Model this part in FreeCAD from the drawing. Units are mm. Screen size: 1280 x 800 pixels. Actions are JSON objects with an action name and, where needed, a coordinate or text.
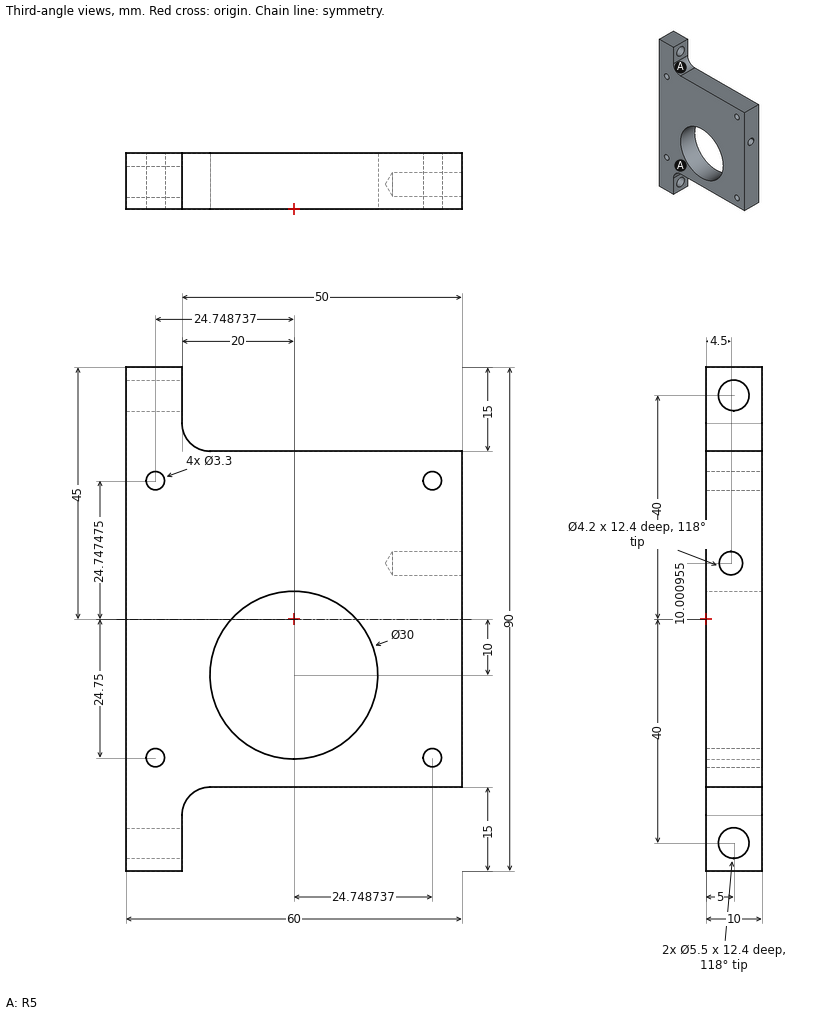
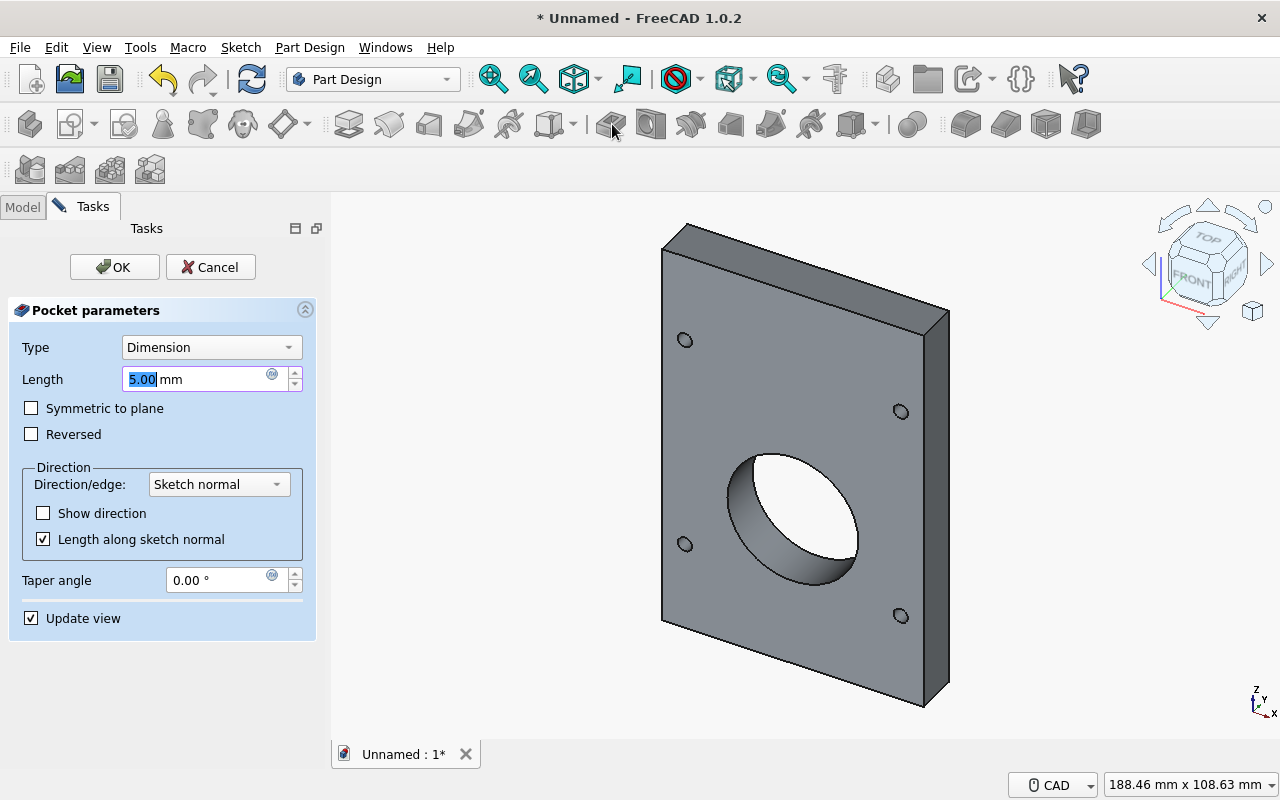
{"action": "left_click", "coordinate": [212, 348]}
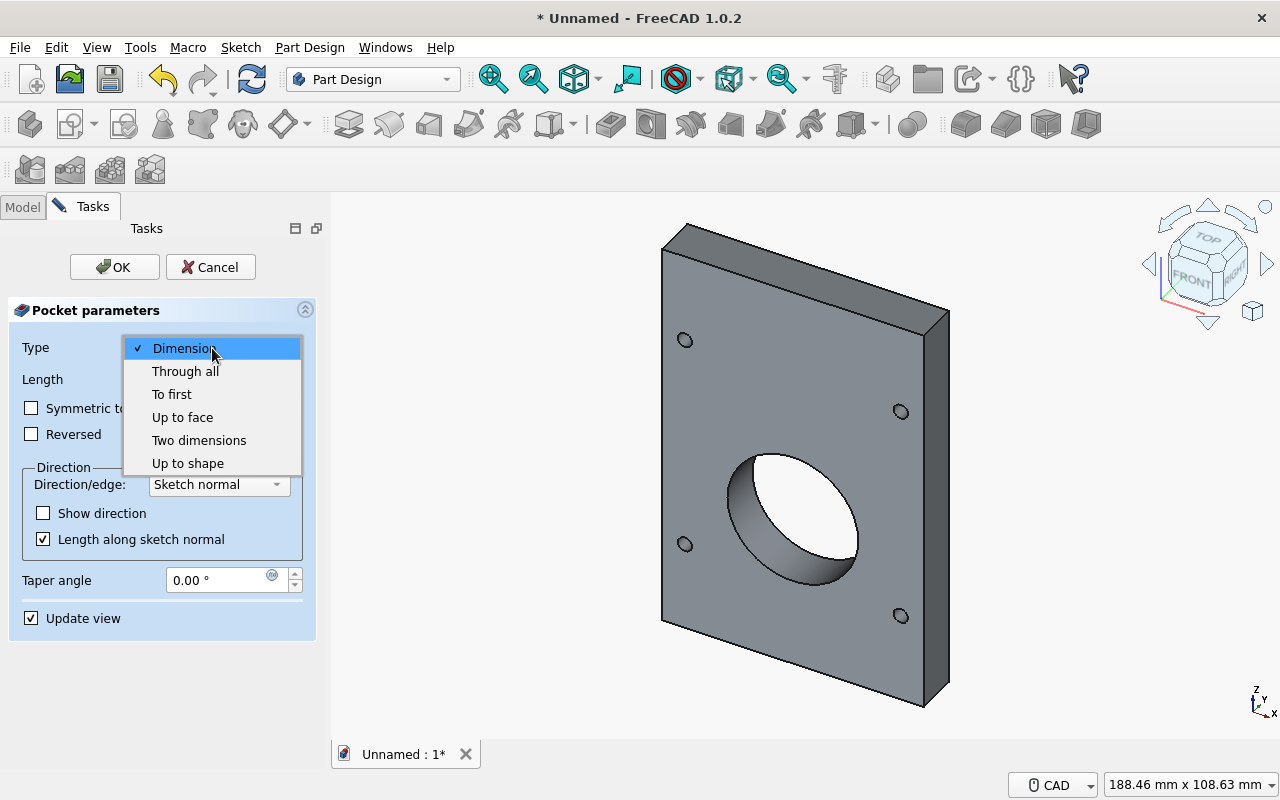
{"action": "left_click", "coordinate": [212, 372]}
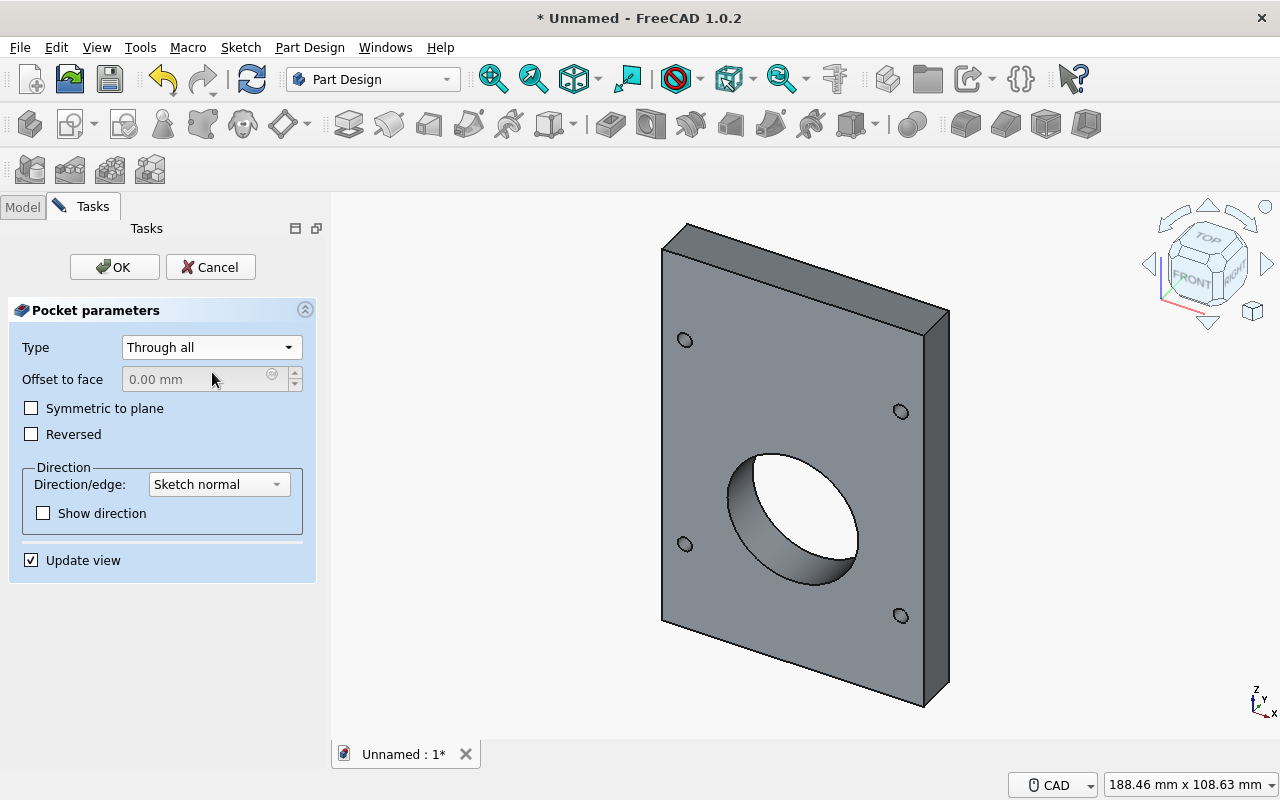
{"action": "left_click", "coordinate": [115, 267]}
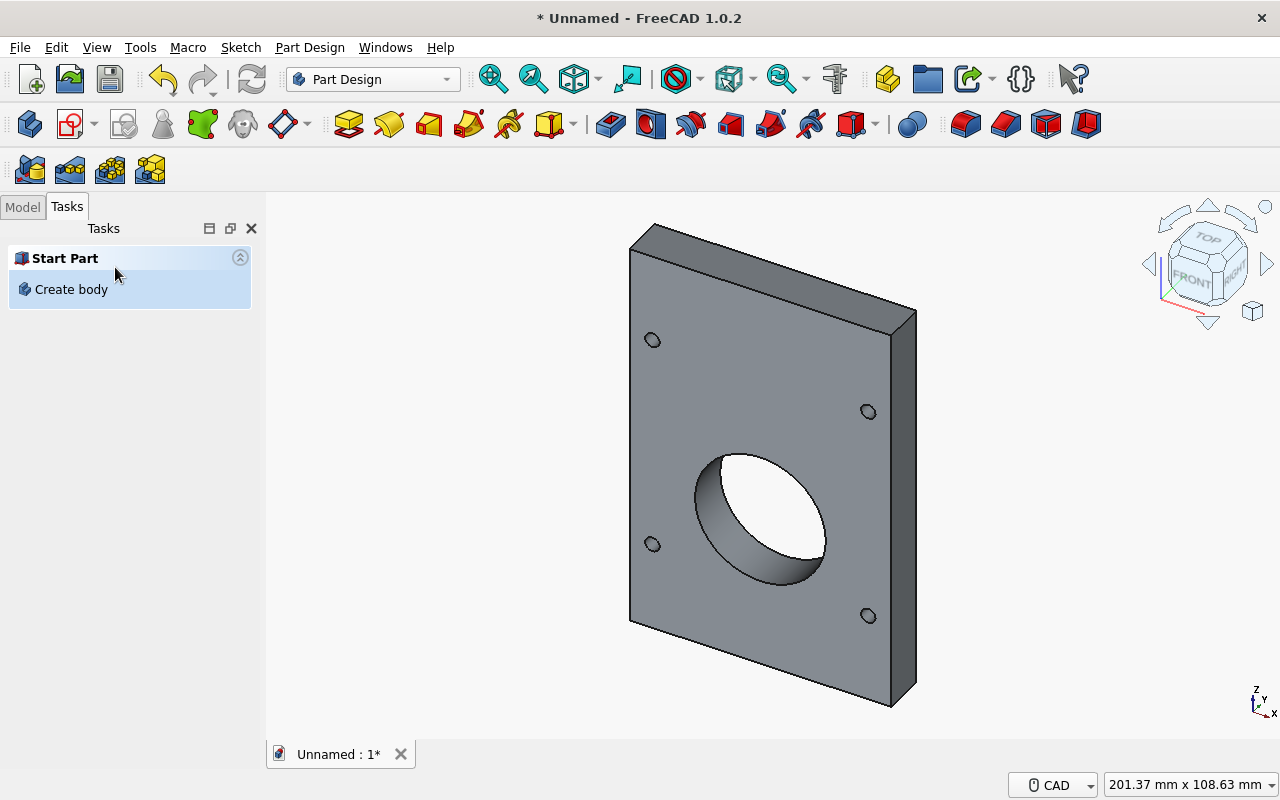
{"action": "left_click", "coordinate": [760, 371]}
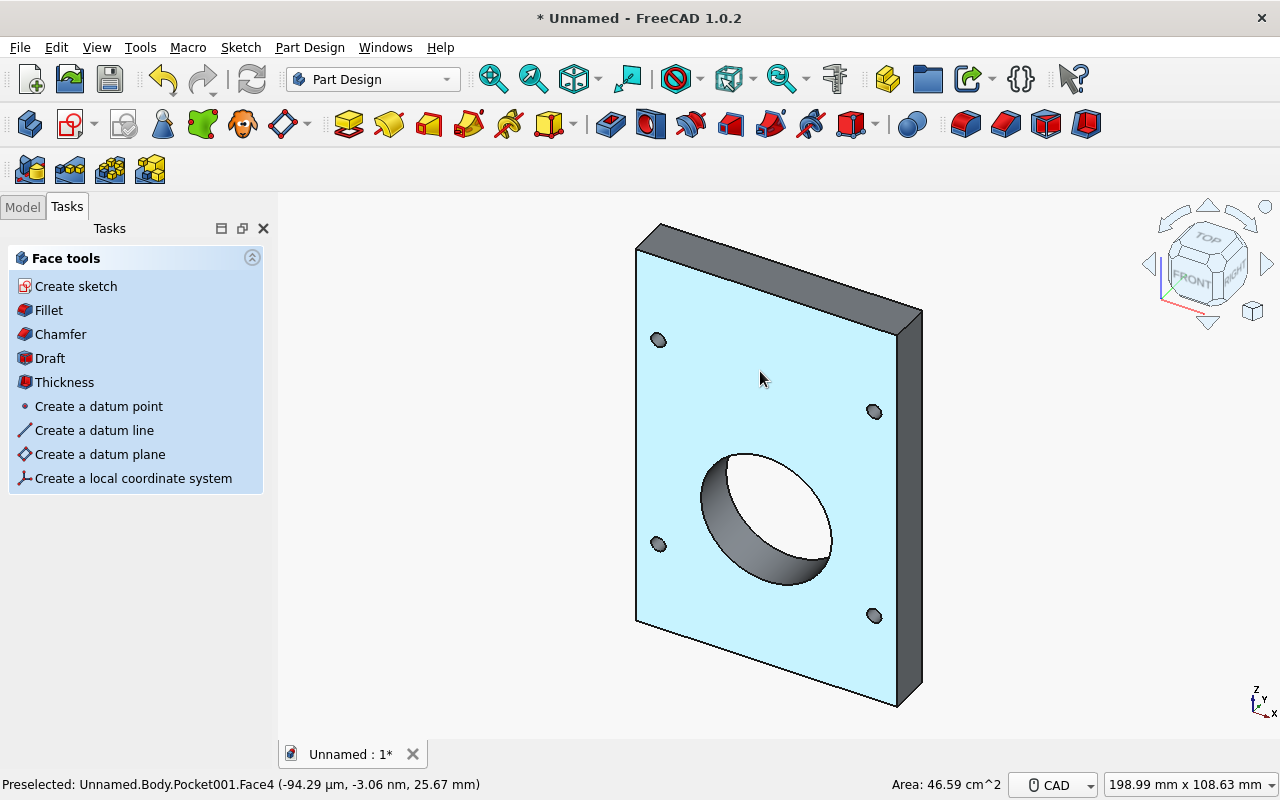
{"action": "left_click", "coordinate": [70, 124]}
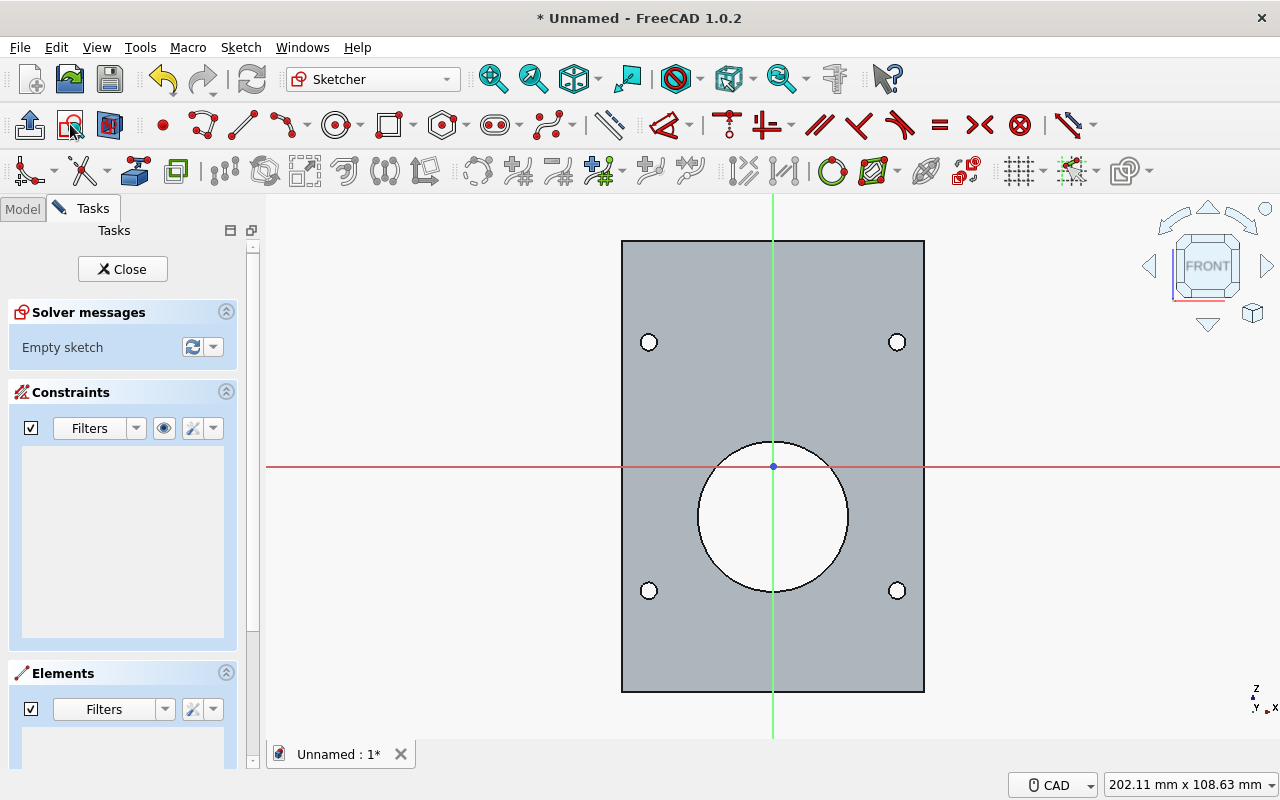
{"action": "scroll", "coordinate": [294, 466], "scroll_direction": "down", "scroll_amount": 1}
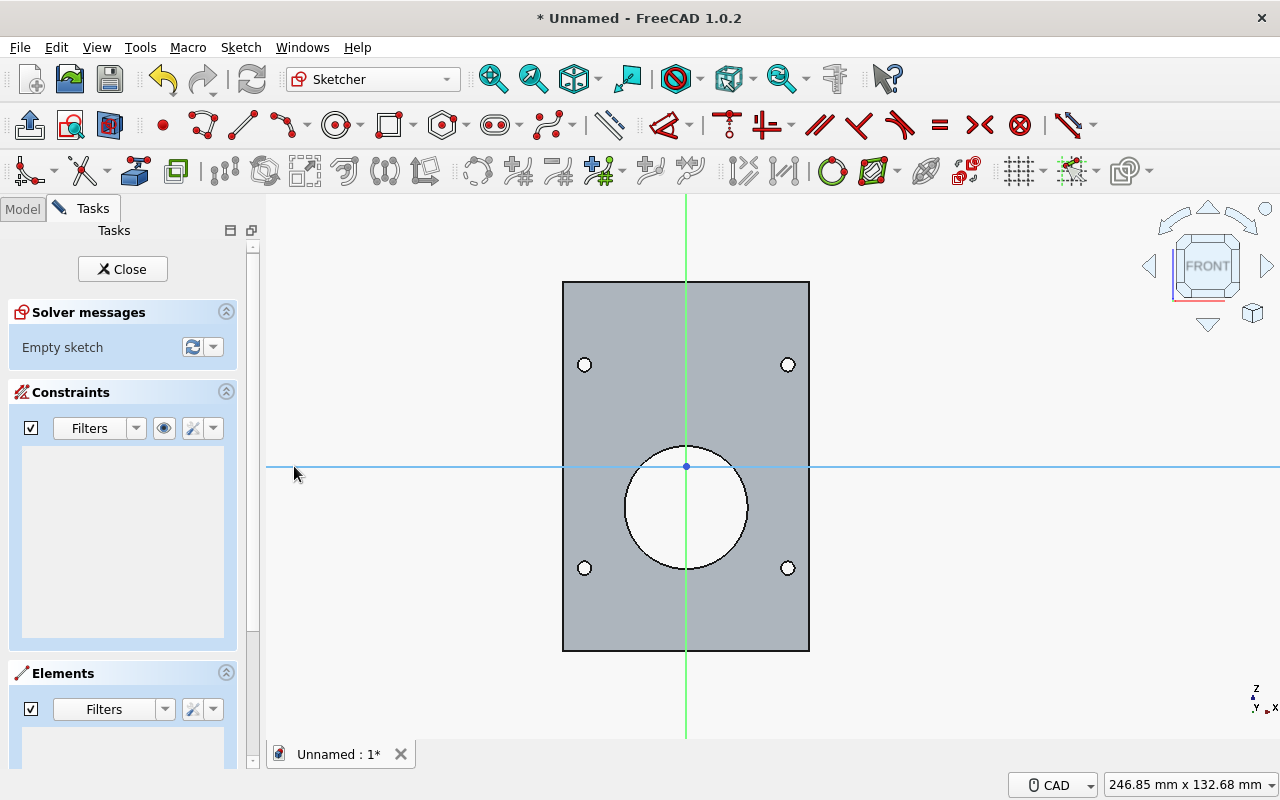
{"action": "left_click", "coordinate": [390, 126]}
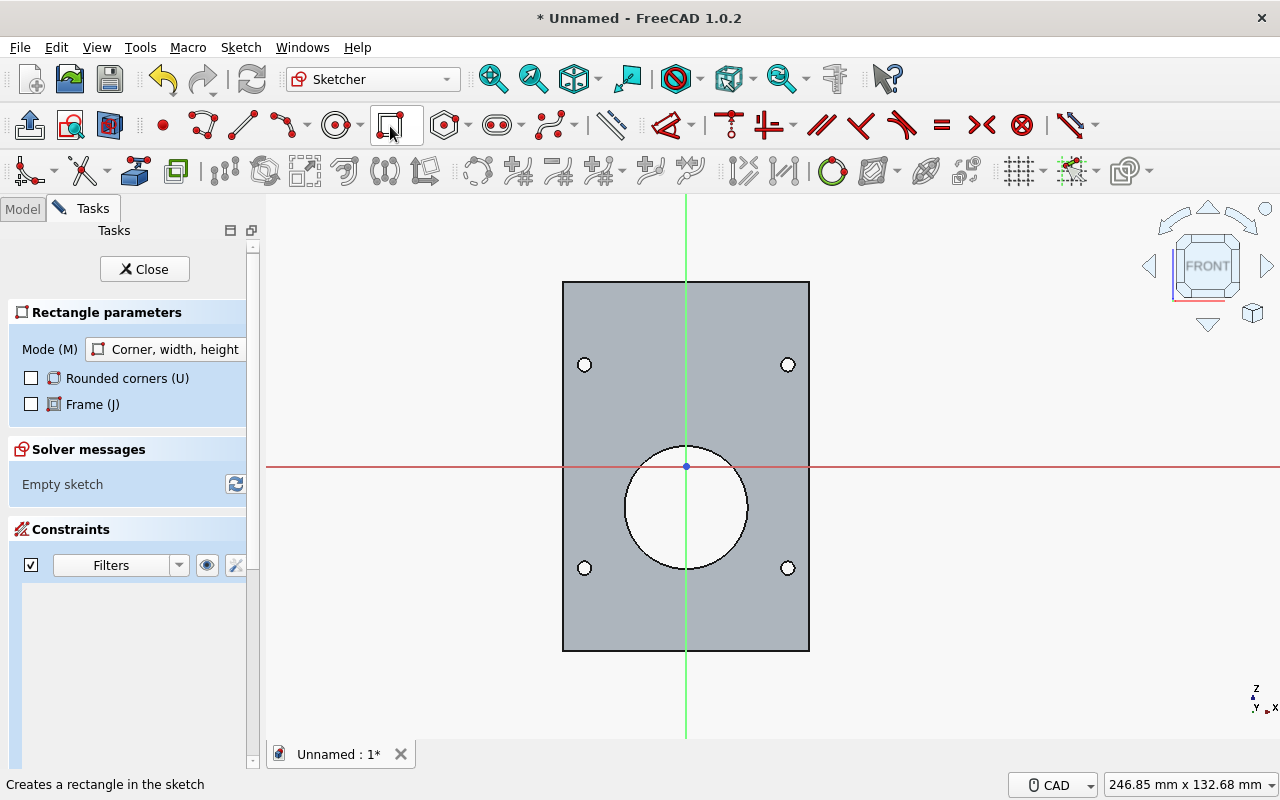
{"action": "left_click", "coordinate": [604, 282]}
{"action": "mouse_move", "coordinate": [809, 343]}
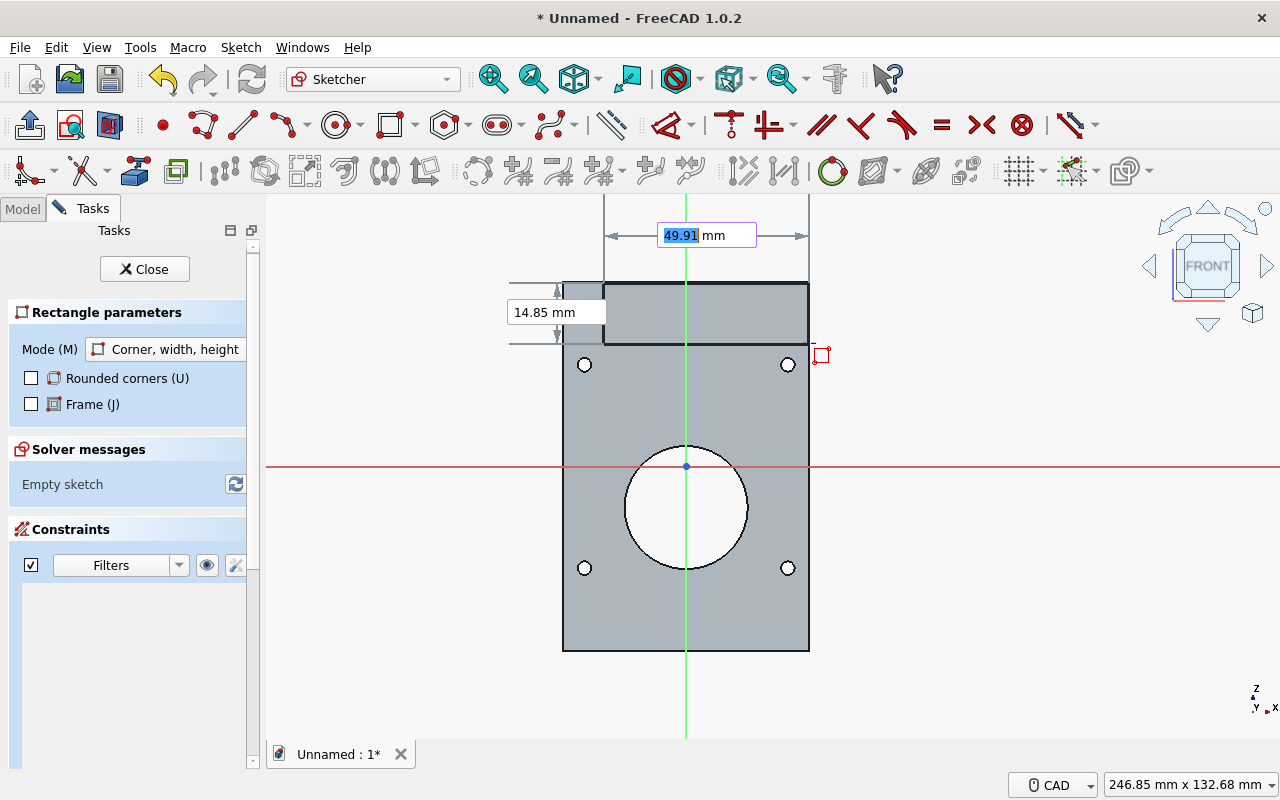
{"action": "type", "text": "50"}
{"action": "key", "text": "Tab"}
{"action": "type", "text": "15"}
{"action": "key", "text": "Return"}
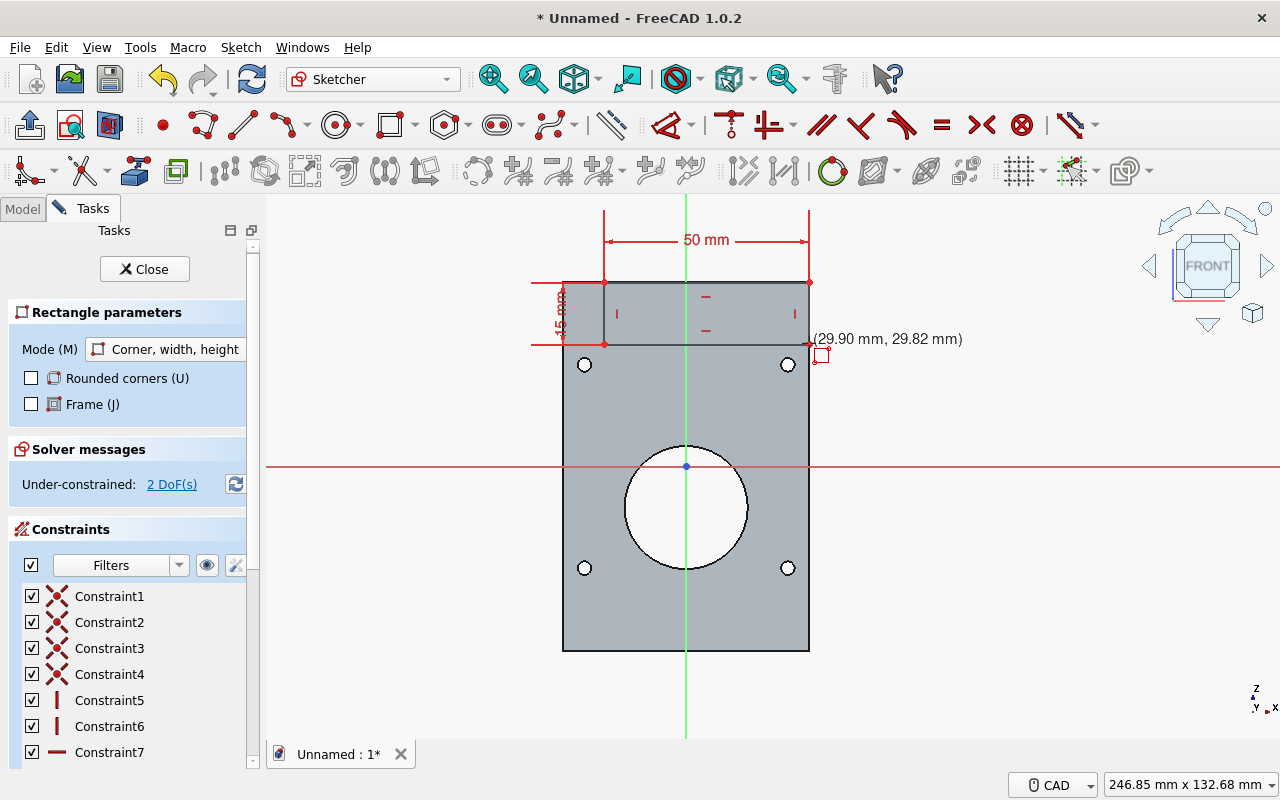
{"action": "left_click", "coordinate": [604, 590]}
{"action": "mouse_move", "coordinate": [809, 651]}